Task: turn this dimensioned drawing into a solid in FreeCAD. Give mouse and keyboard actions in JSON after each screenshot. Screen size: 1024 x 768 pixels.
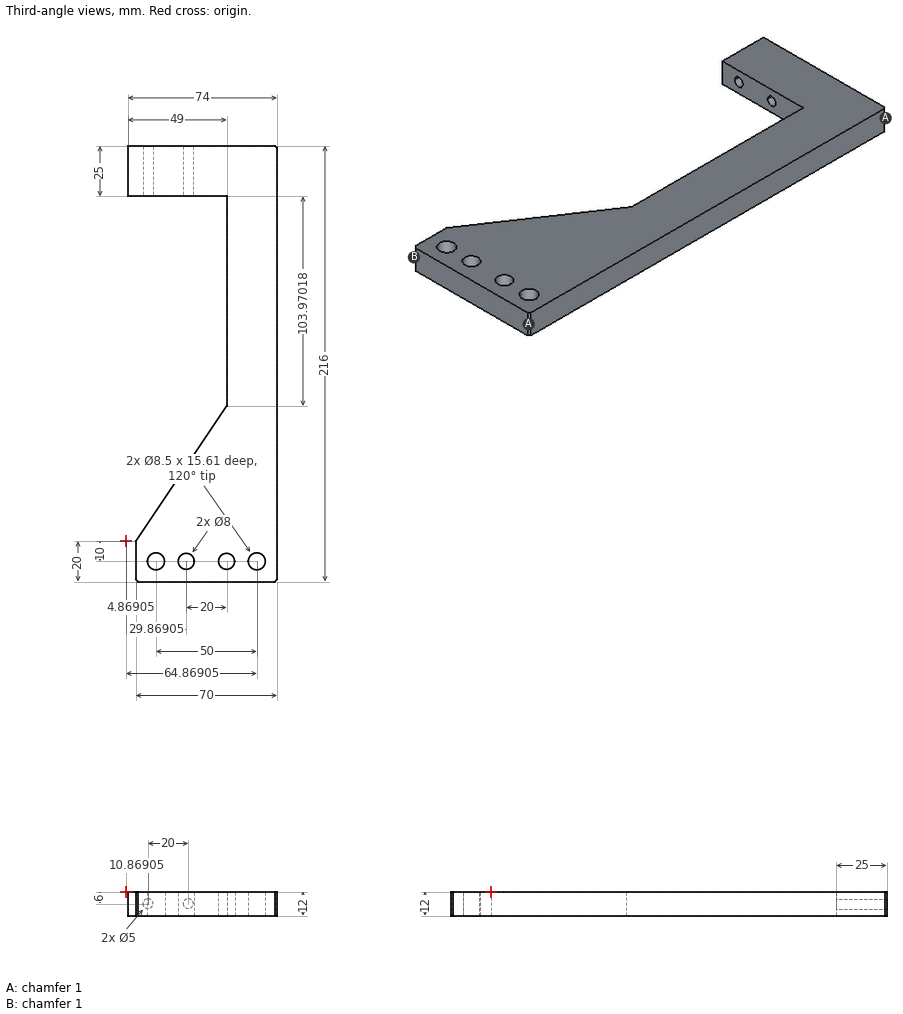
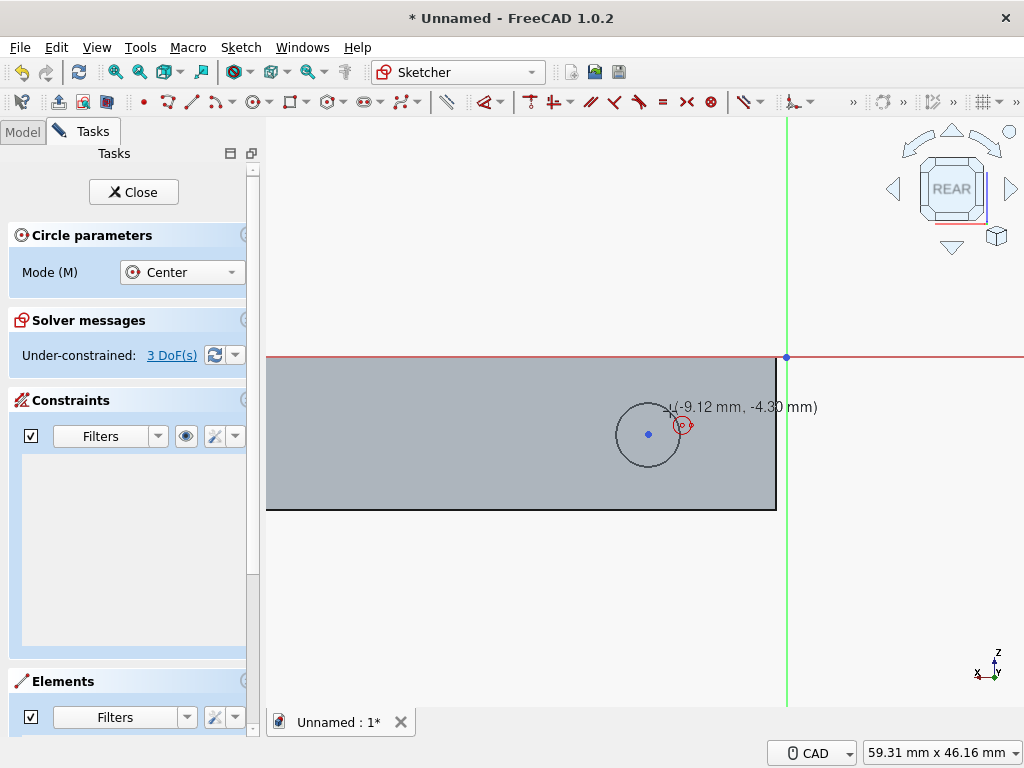
{"action": "left_click", "coordinate": [392, 434]}
{"action": "left_click", "coordinate": [415, 411]}
{"action": "key", "text": "Escape"}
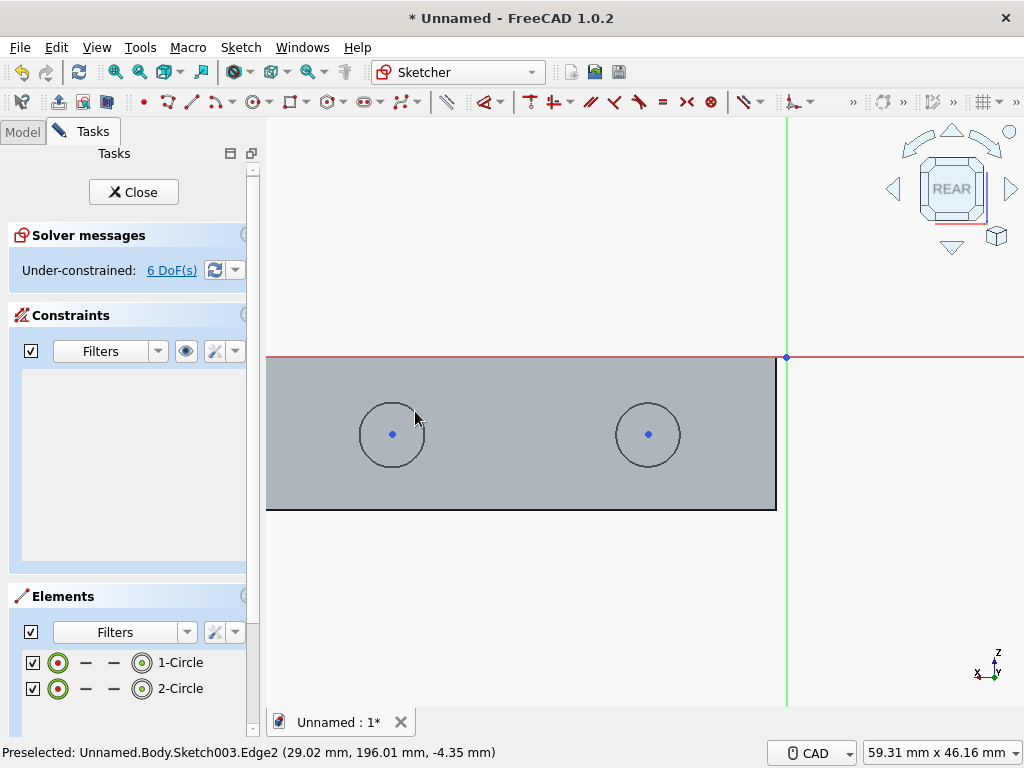
{"action": "left_click", "coordinate": [670, 412]}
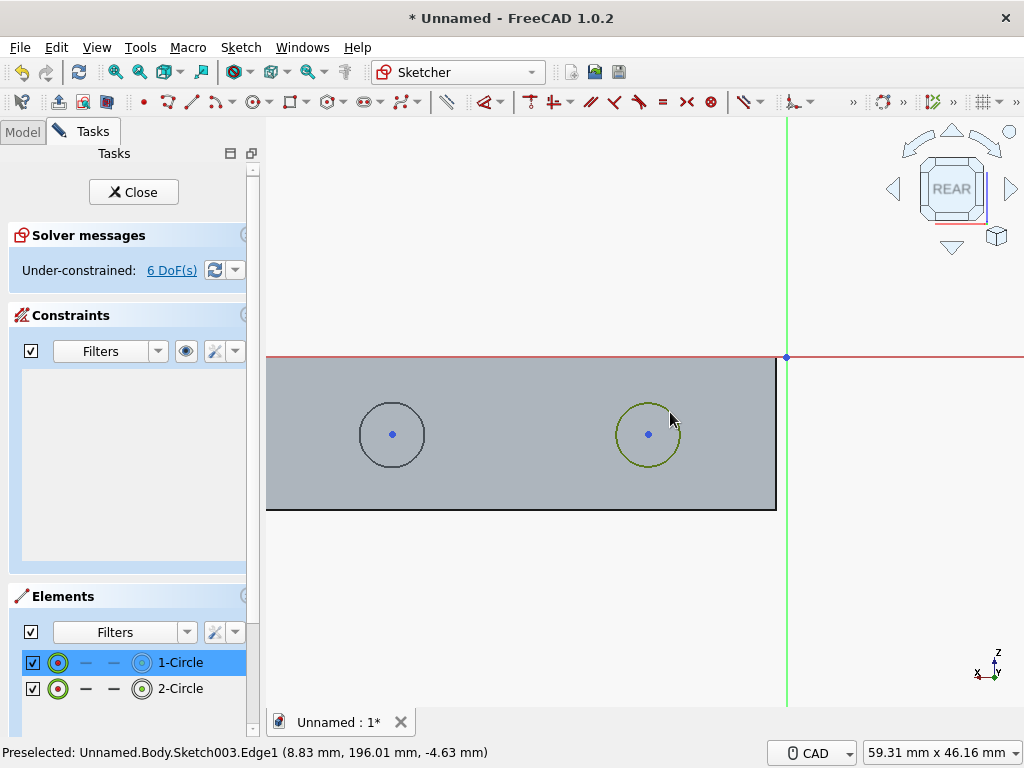
{"action": "left_click", "coordinate": [415, 412]}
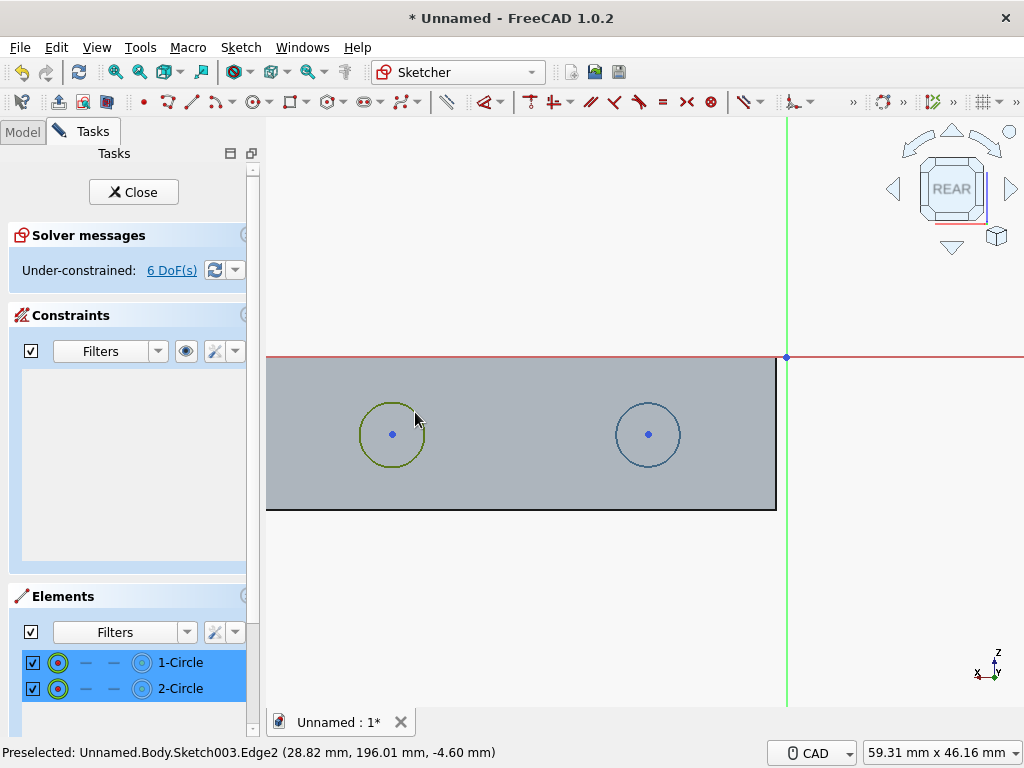
{"action": "key", "text": "e"}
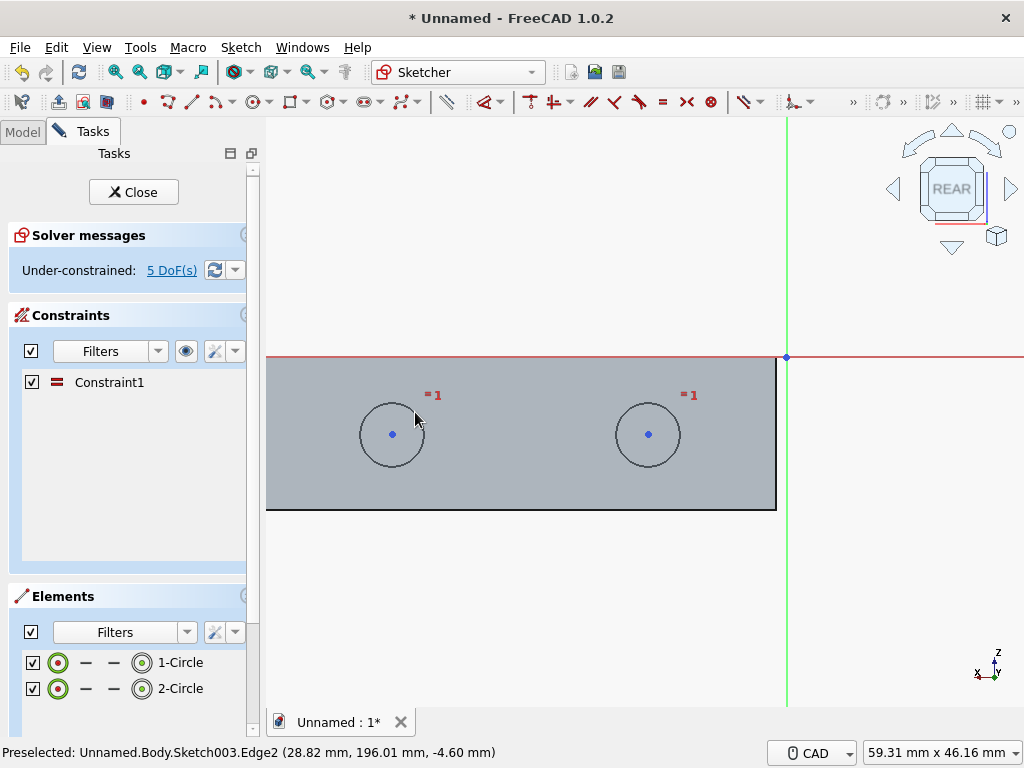
{"action": "key", "text": "d"}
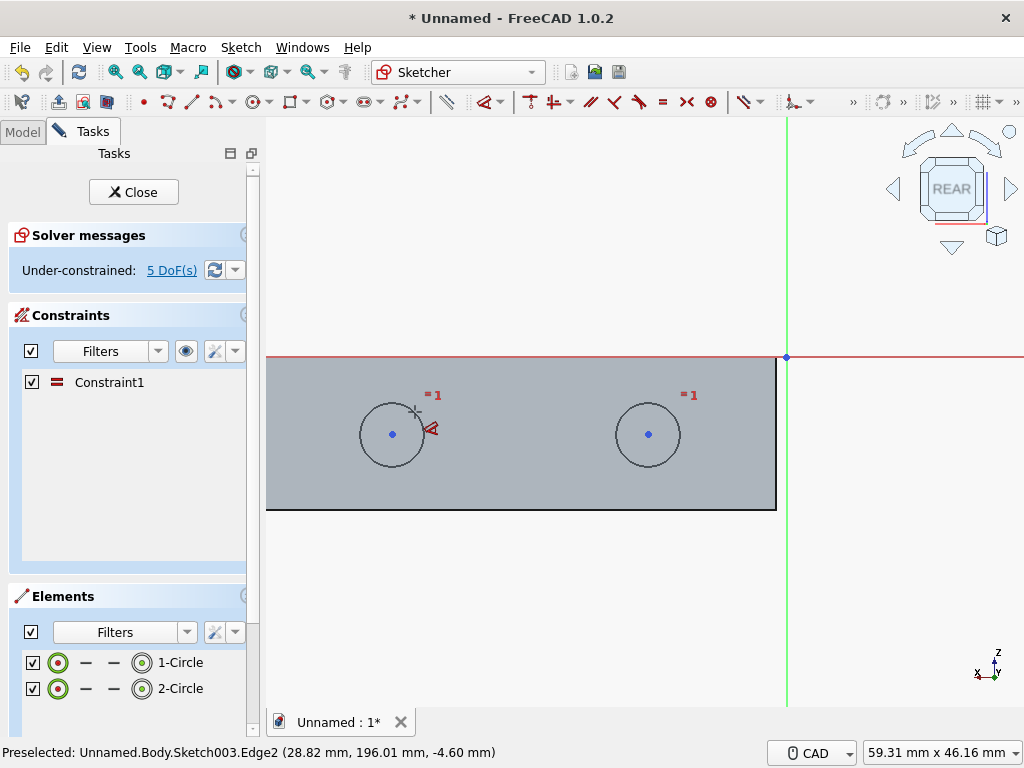
{"action": "left_click", "coordinate": [670, 412]}
{"action": "left_click", "coordinate": [692, 389]}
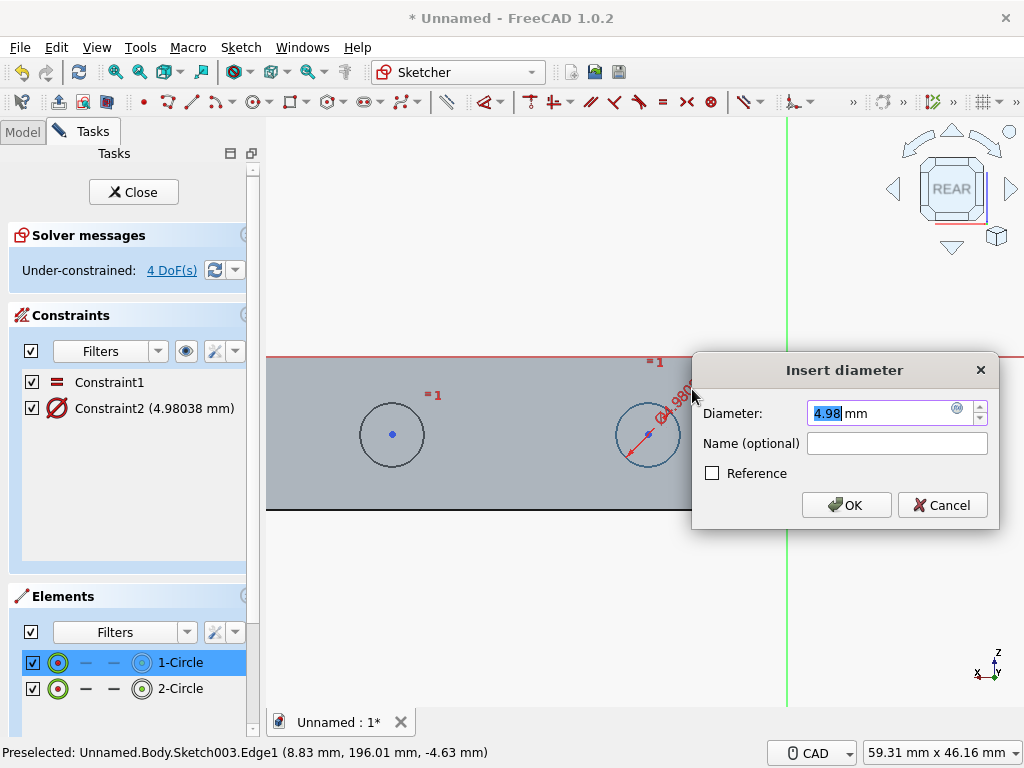
{"action": "type", "text": "5"}
{"action": "key", "text": "Return"}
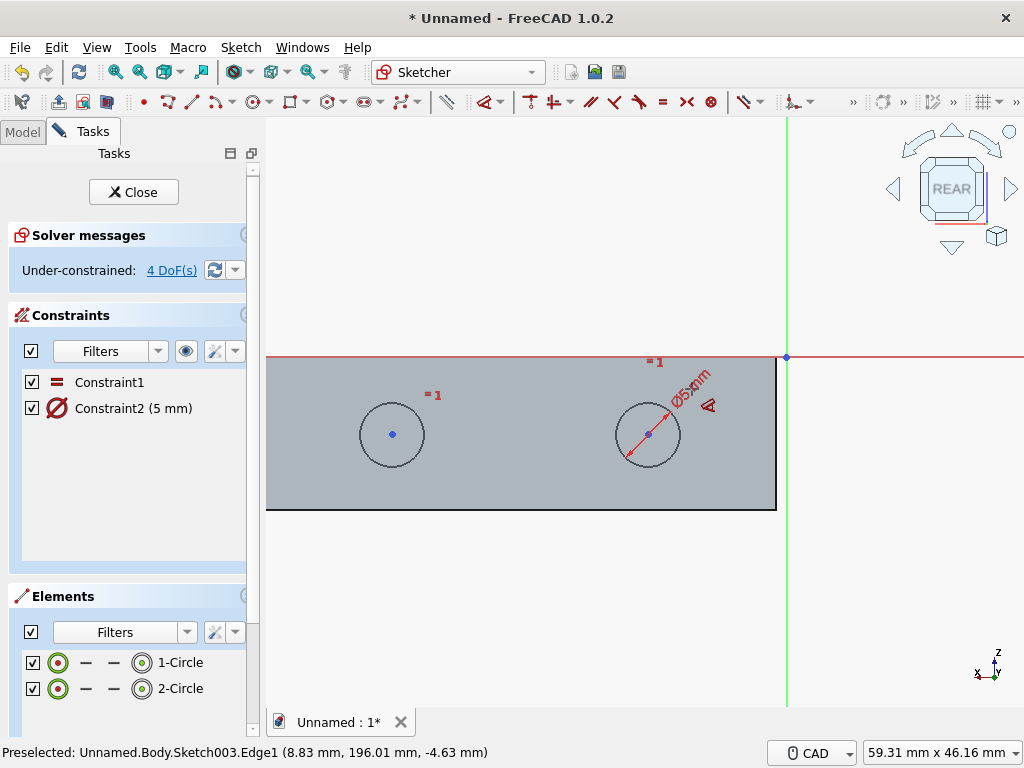
{"action": "left_click", "coordinate": [648, 435]}
{"action": "left_click", "coordinate": [821, 396]}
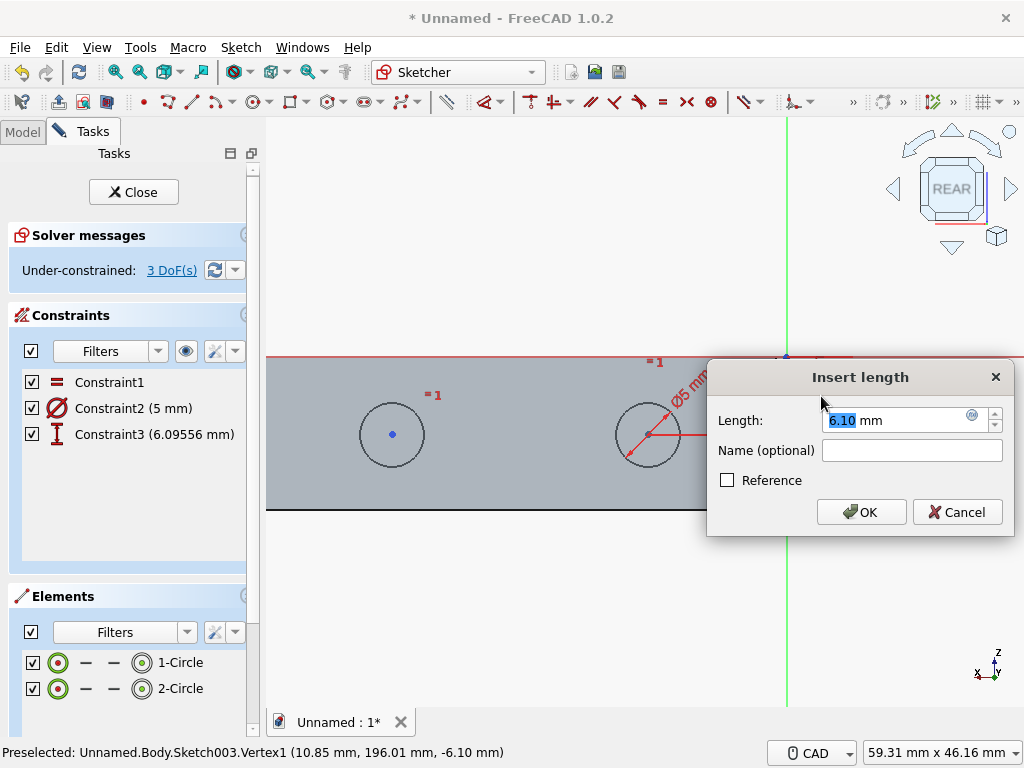
{"action": "type", "text": "6"}
{"action": "key", "text": "Return"}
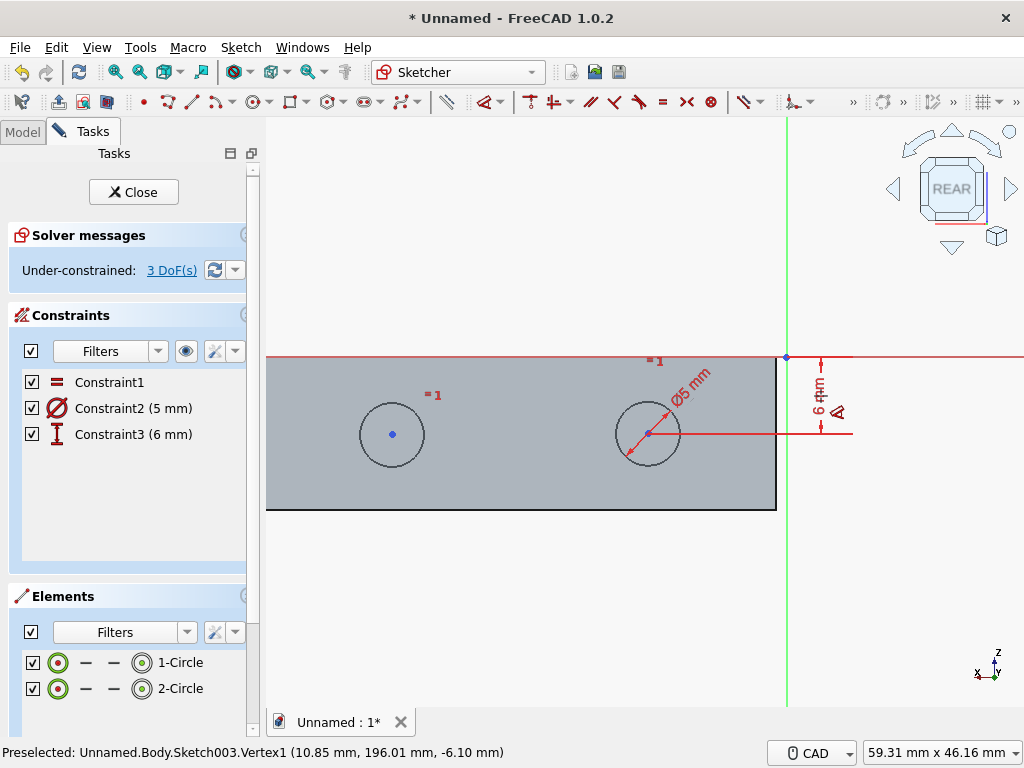
{"action": "left_click", "coordinate": [392, 435]}
{"action": "left_click", "coordinate": [821, 423]}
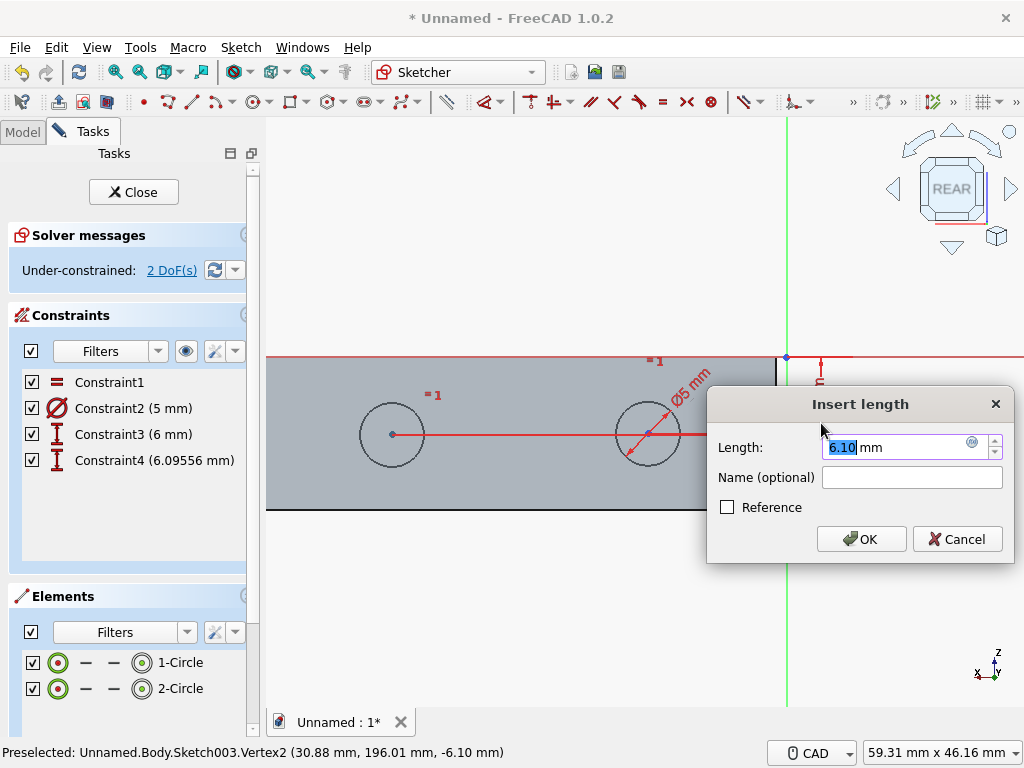
{"action": "type", "text": "6"}
{"action": "key", "text": "Return"}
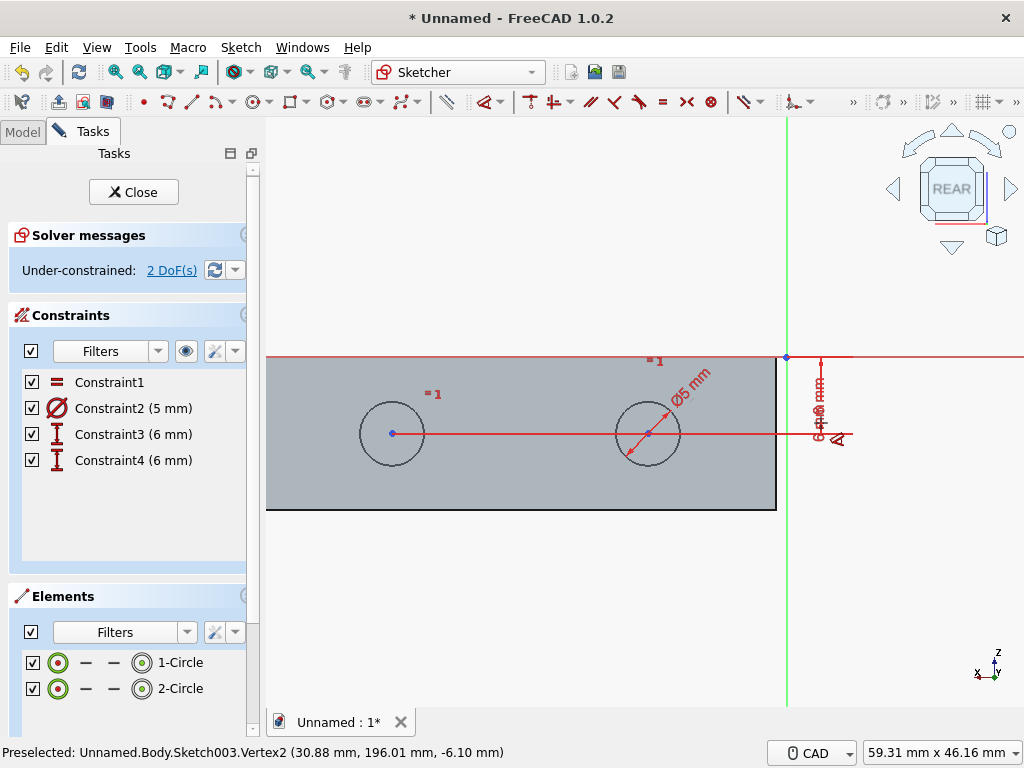
{"action": "left_click", "coordinate": [648, 434]}